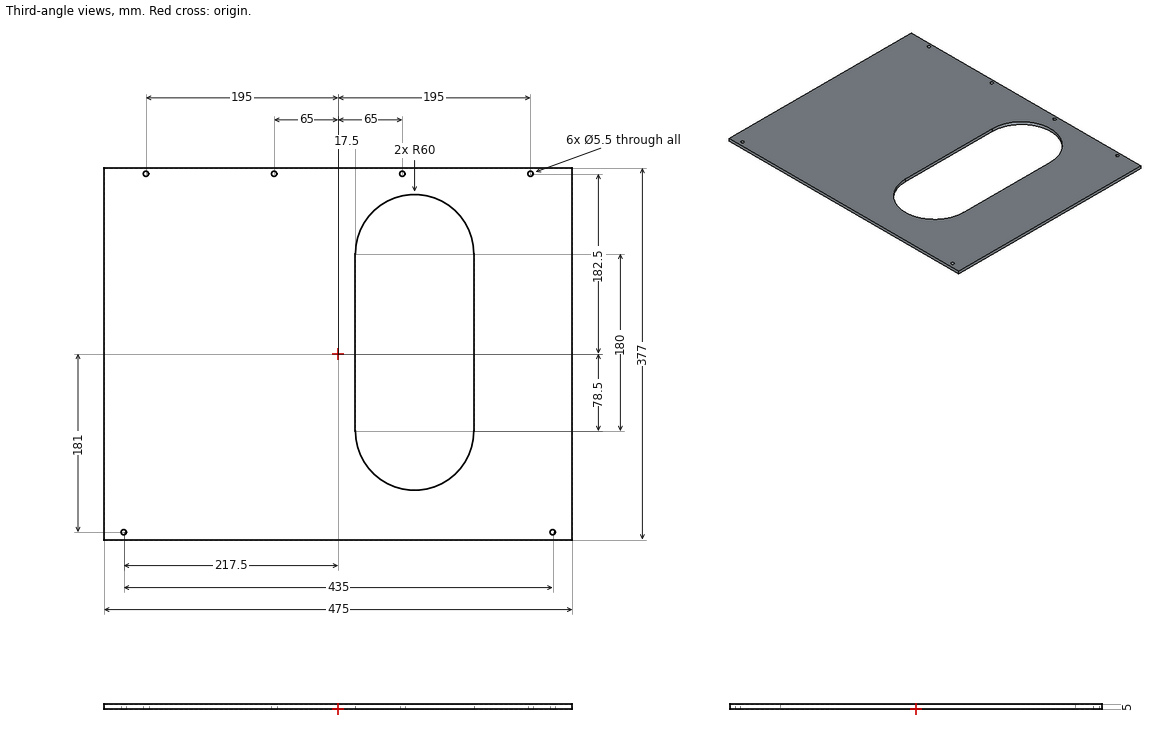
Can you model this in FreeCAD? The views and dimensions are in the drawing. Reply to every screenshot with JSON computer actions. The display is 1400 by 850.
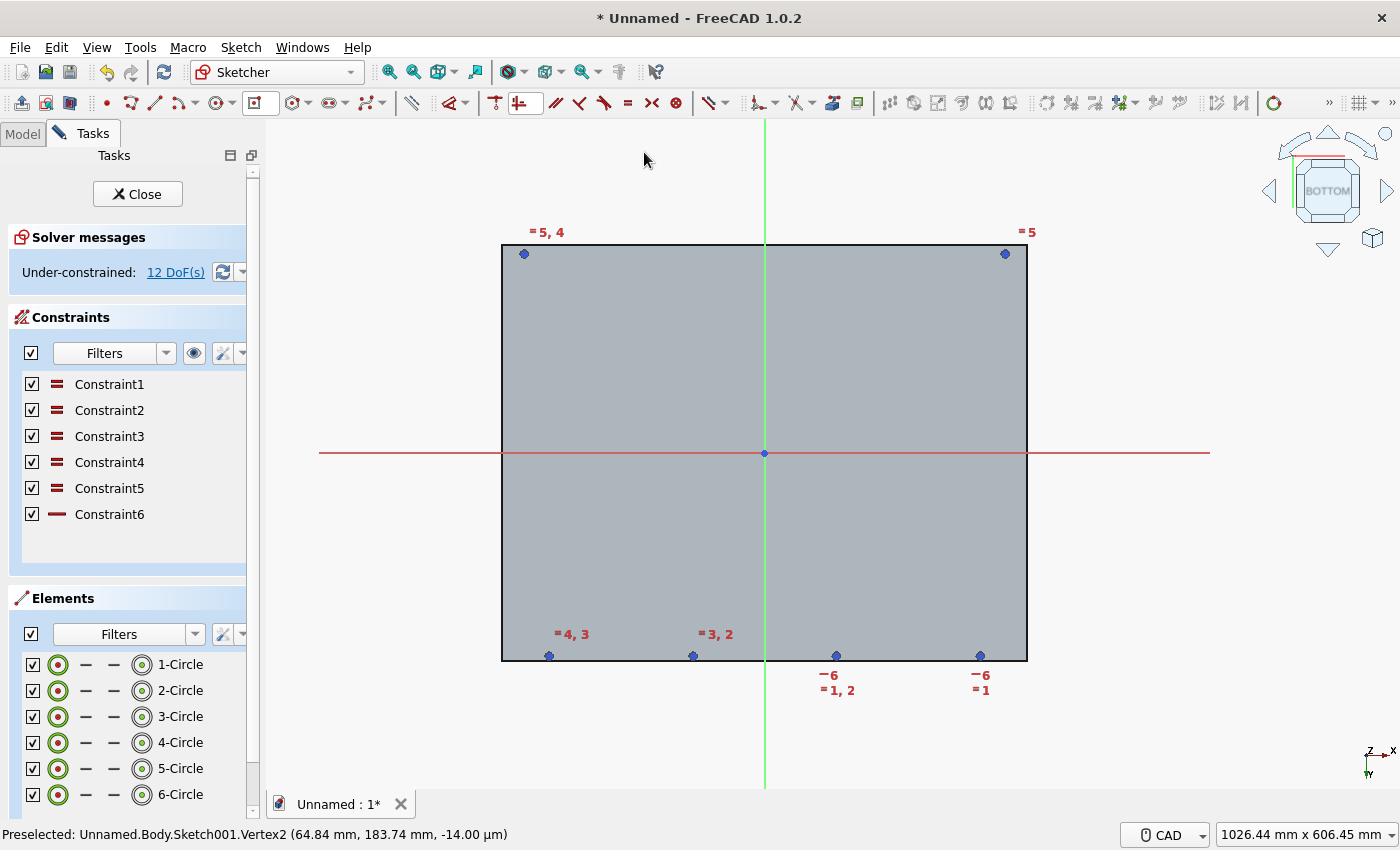
{"action": "left_click", "coordinate": [836, 656]}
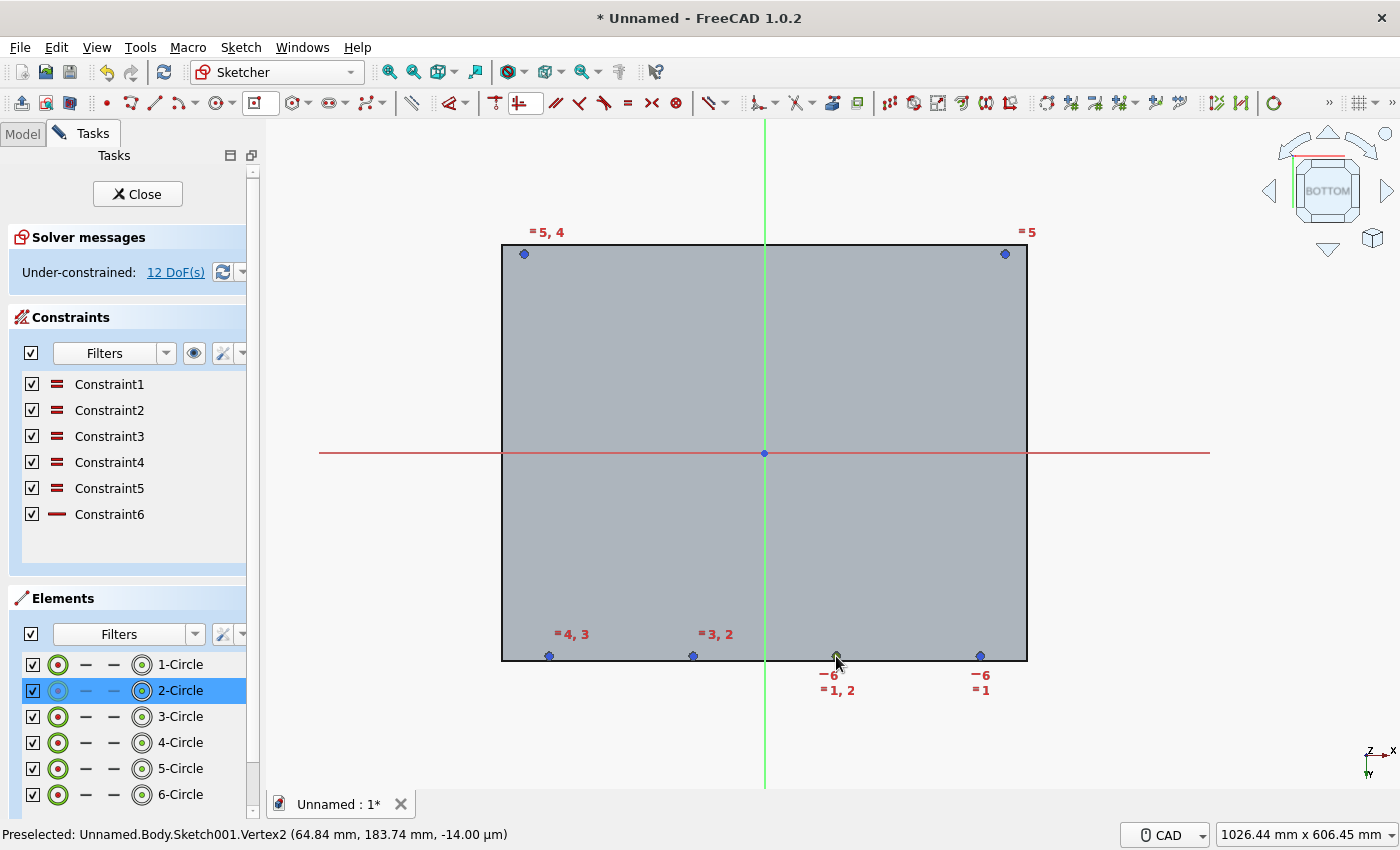
{"action": "left_click", "coordinate": [693, 656]}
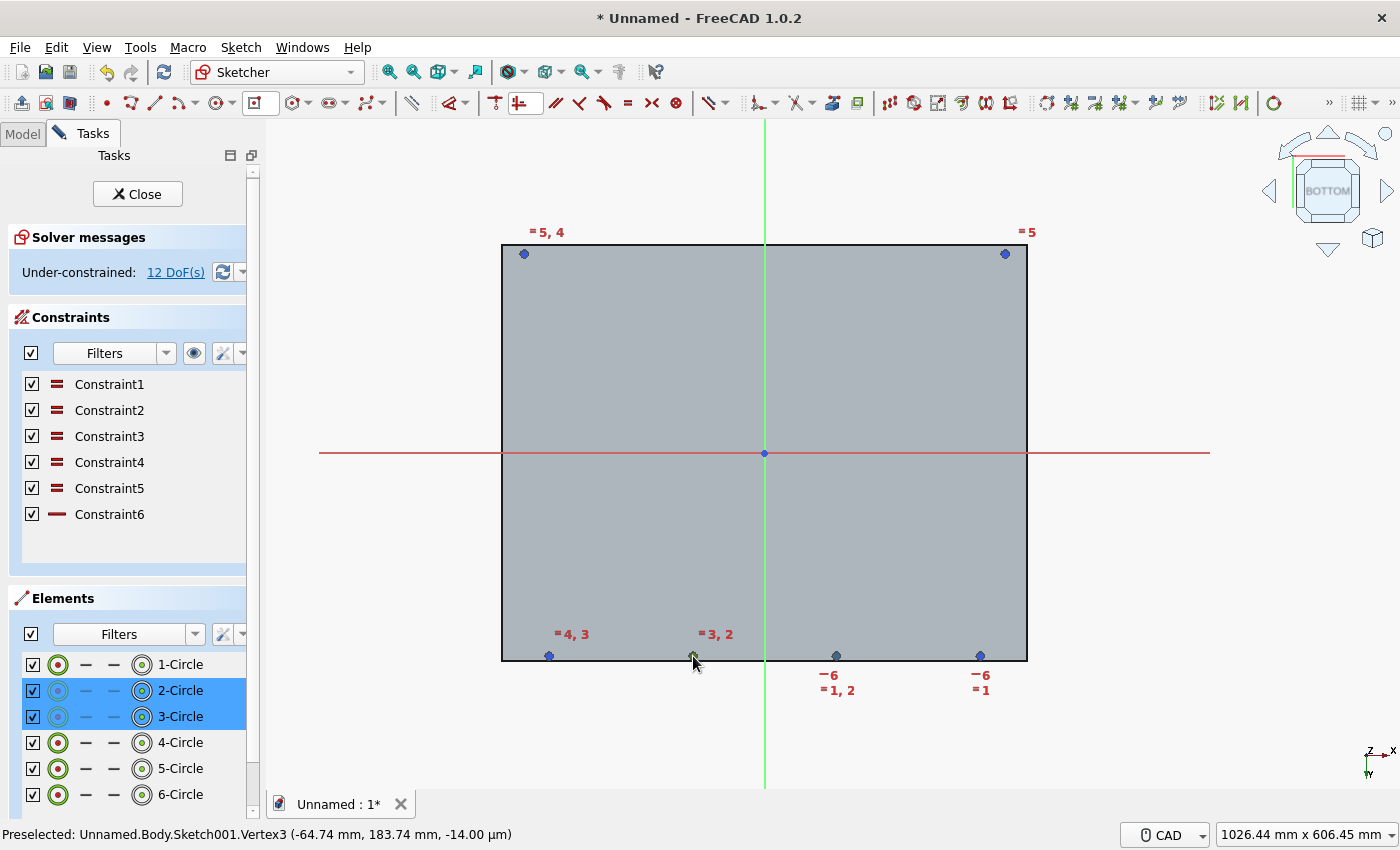
{"action": "left_click", "coordinate": [538, 104]}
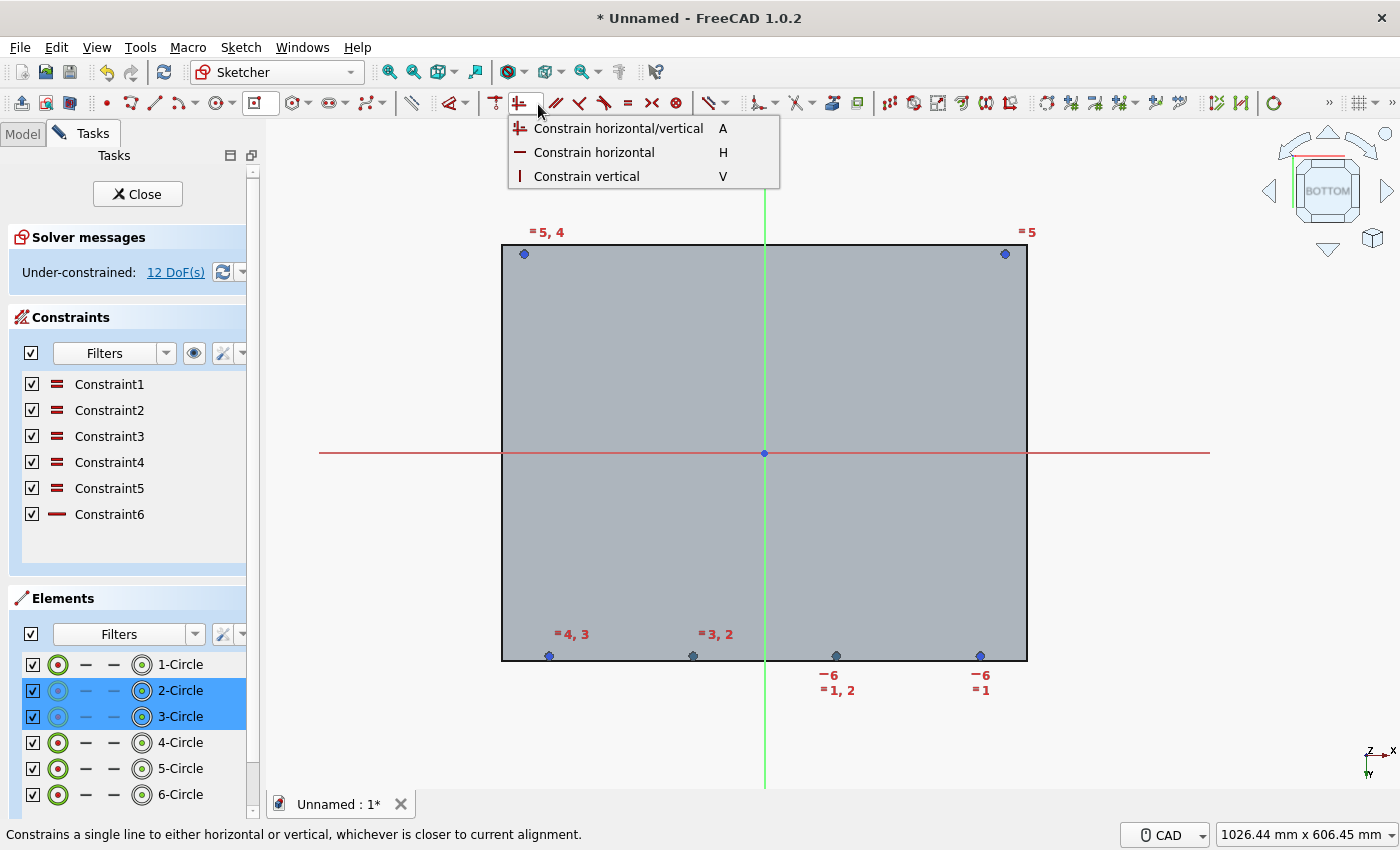
{"action": "left_click", "coordinate": [644, 152]}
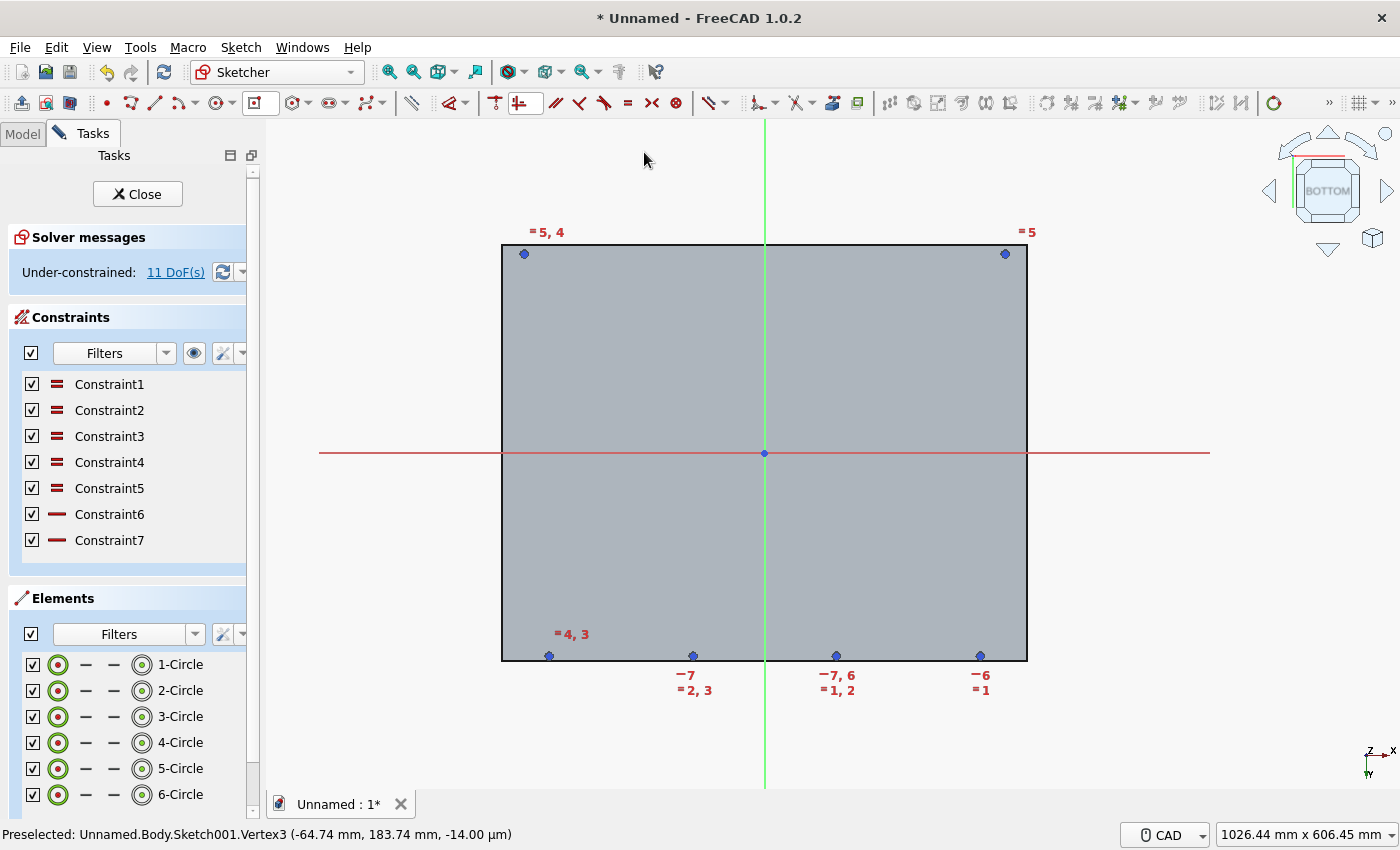
{"action": "left_click", "coordinate": [693, 656]}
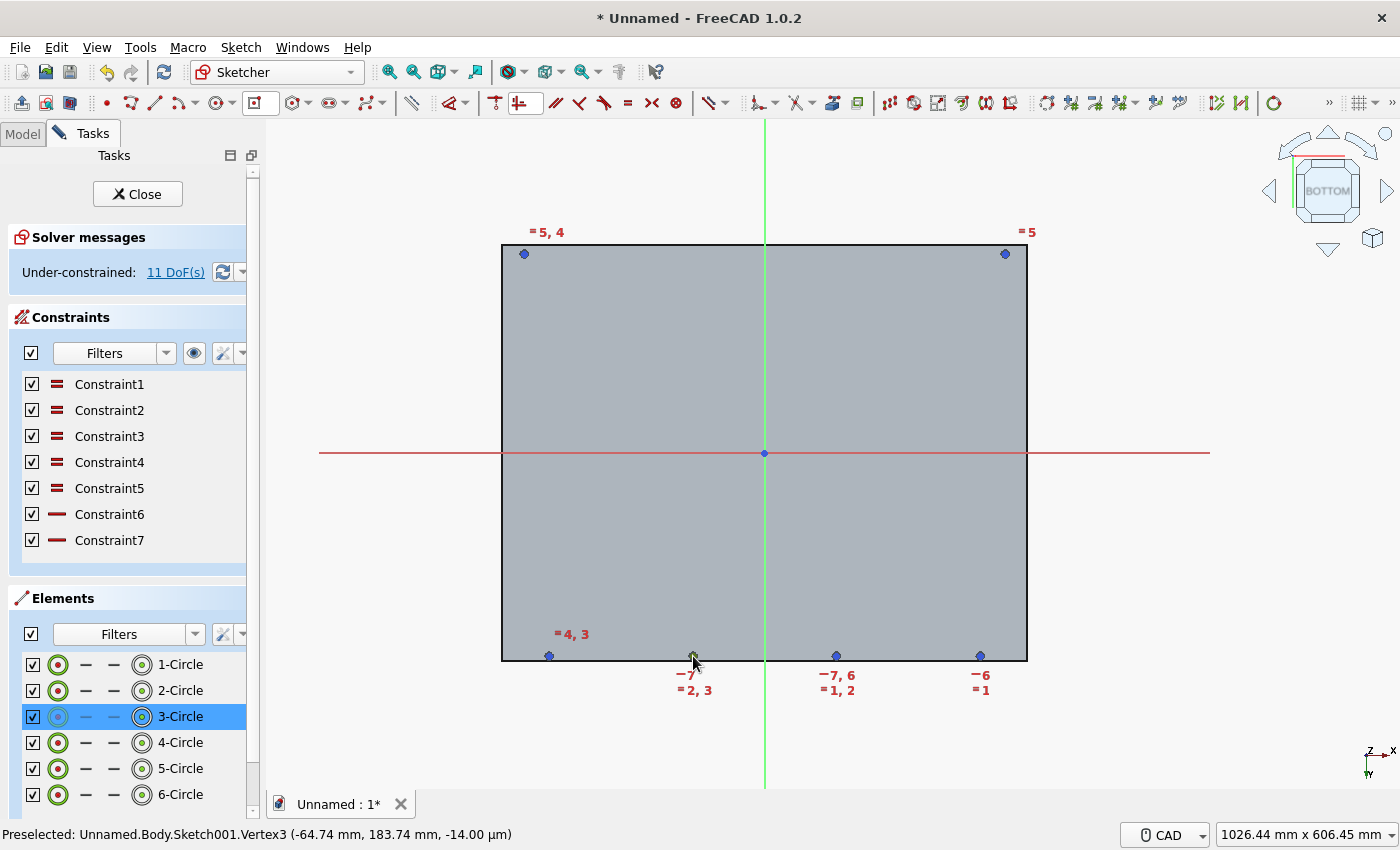
{"action": "left_click", "coordinate": [549, 656]}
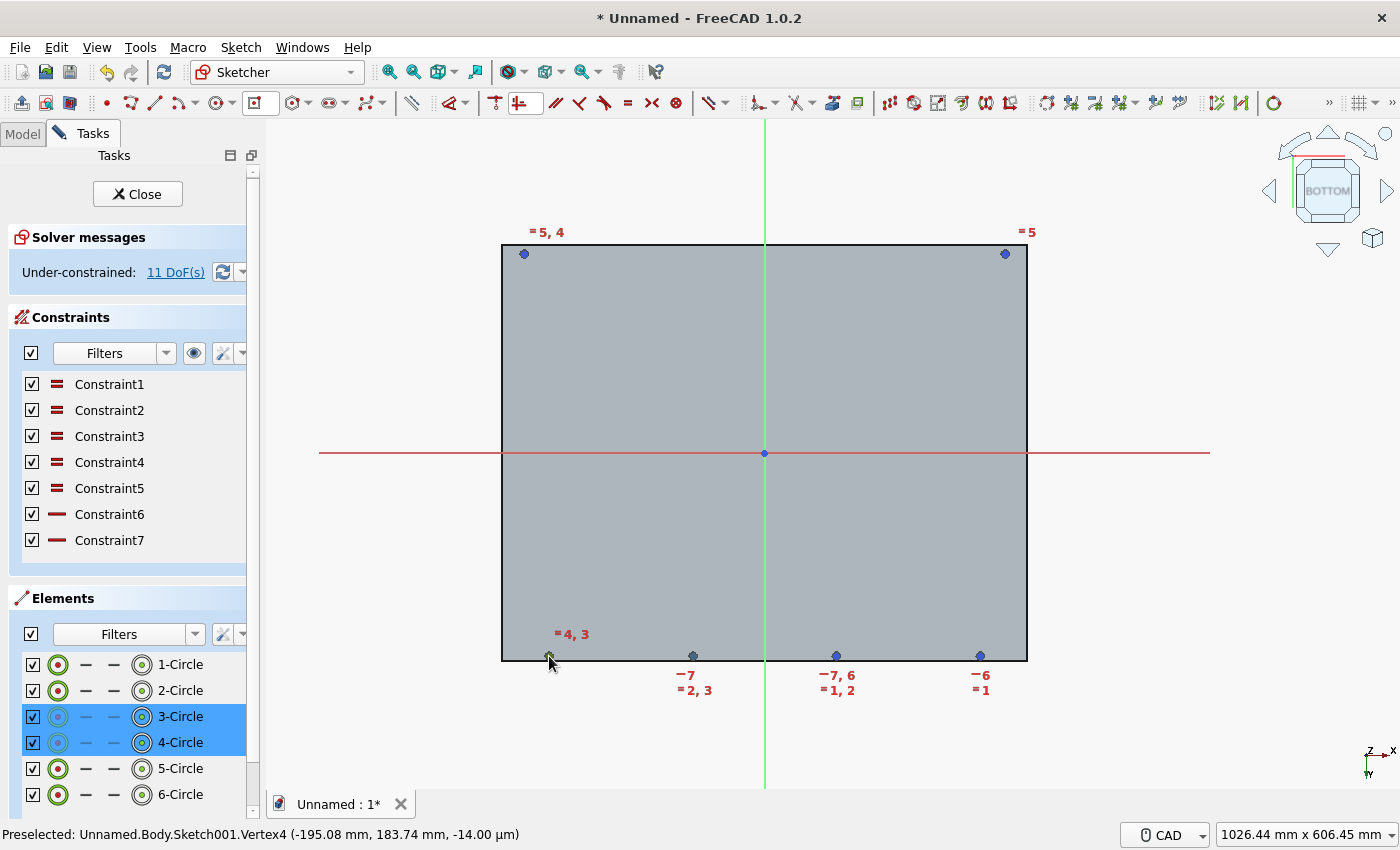
{"action": "key", "text": "h"}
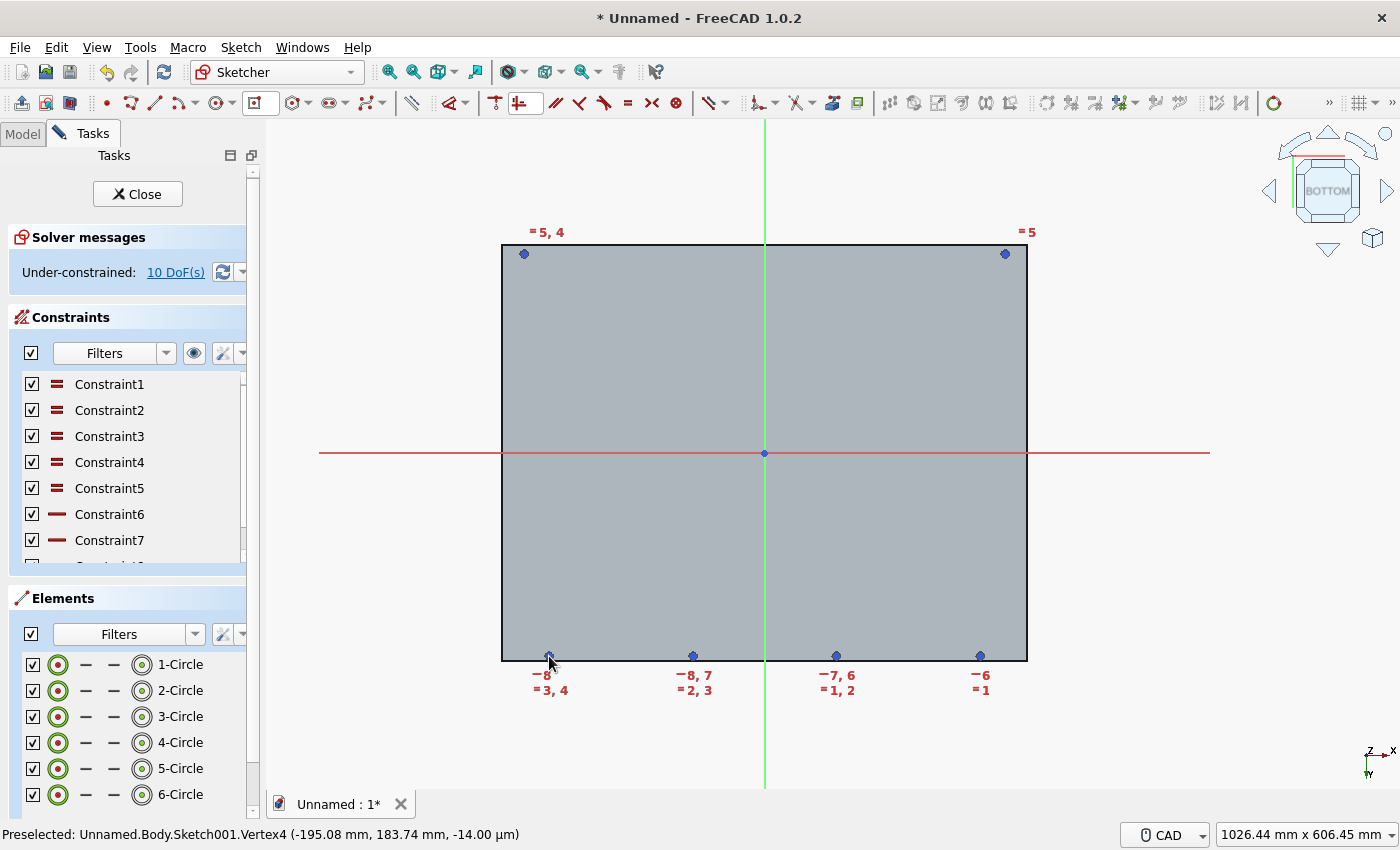
{"action": "left_click", "coordinate": [524, 254]}